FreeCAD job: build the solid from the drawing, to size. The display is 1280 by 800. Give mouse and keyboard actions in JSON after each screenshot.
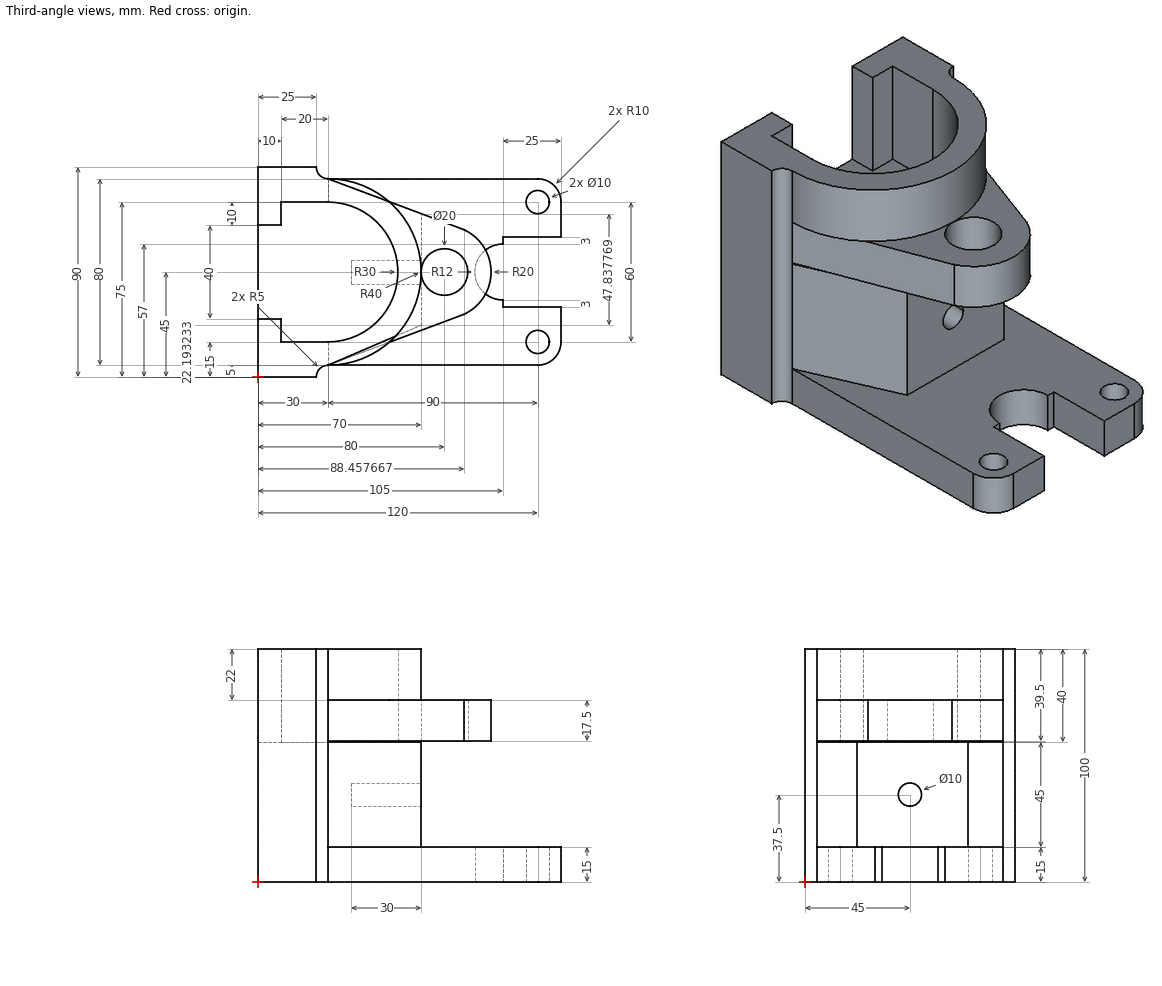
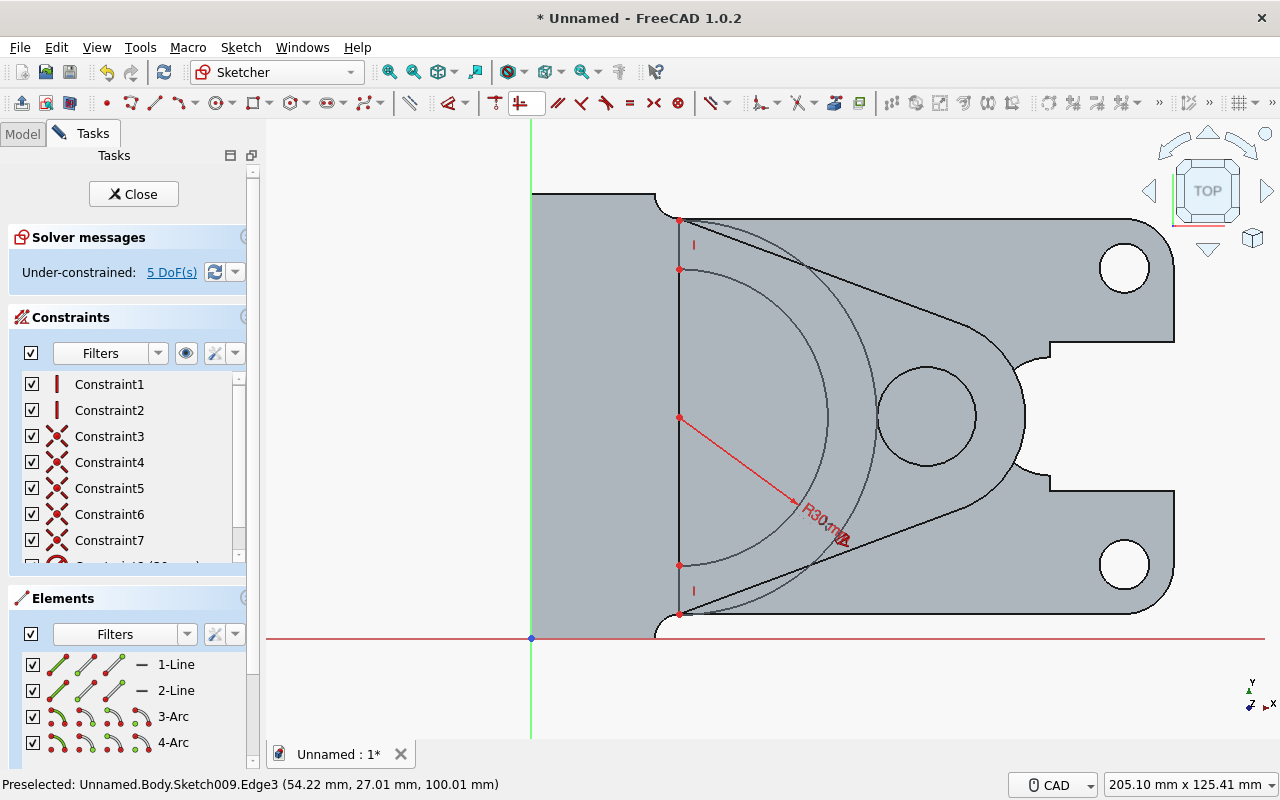
{"action": "left_click", "coordinate": [839, 534]}
{"action": "left_click", "coordinate": [865, 553]}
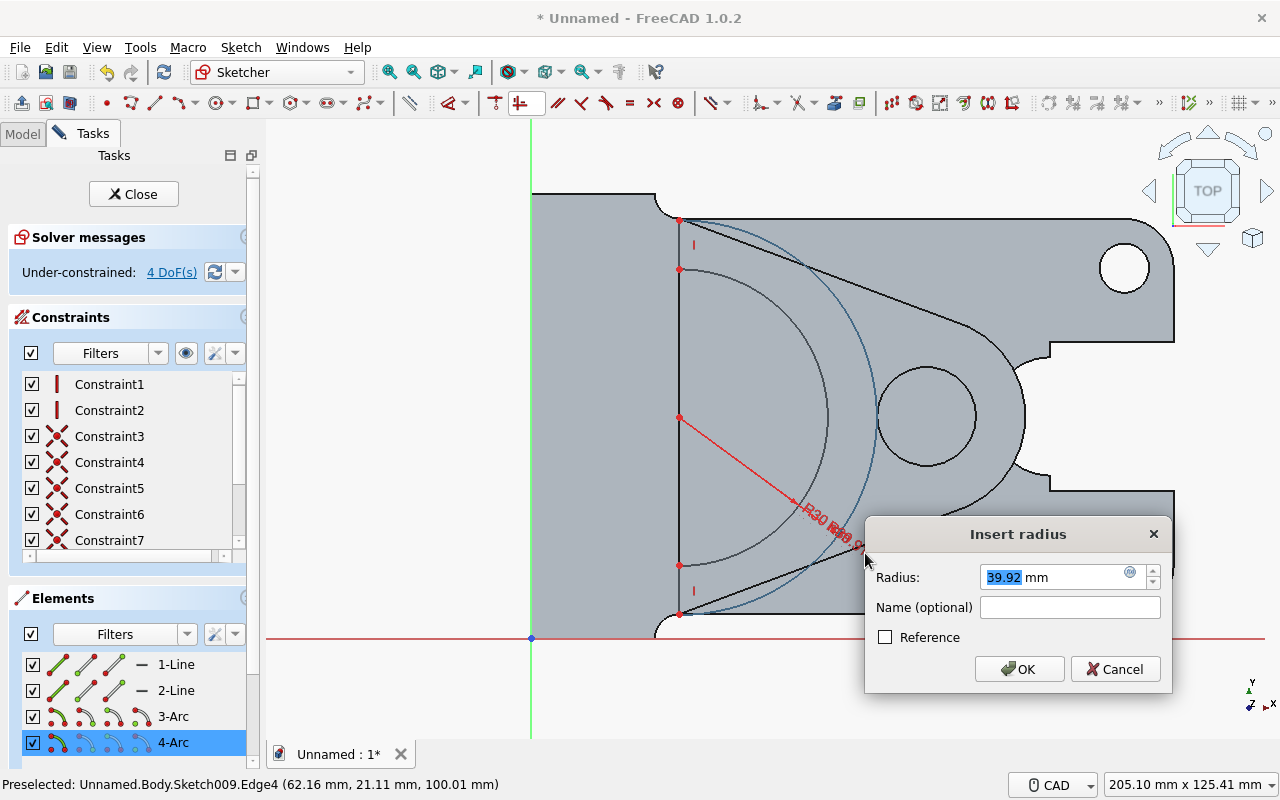
{"action": "type", "text": "40"}
{"action": "key", "text": "Return"}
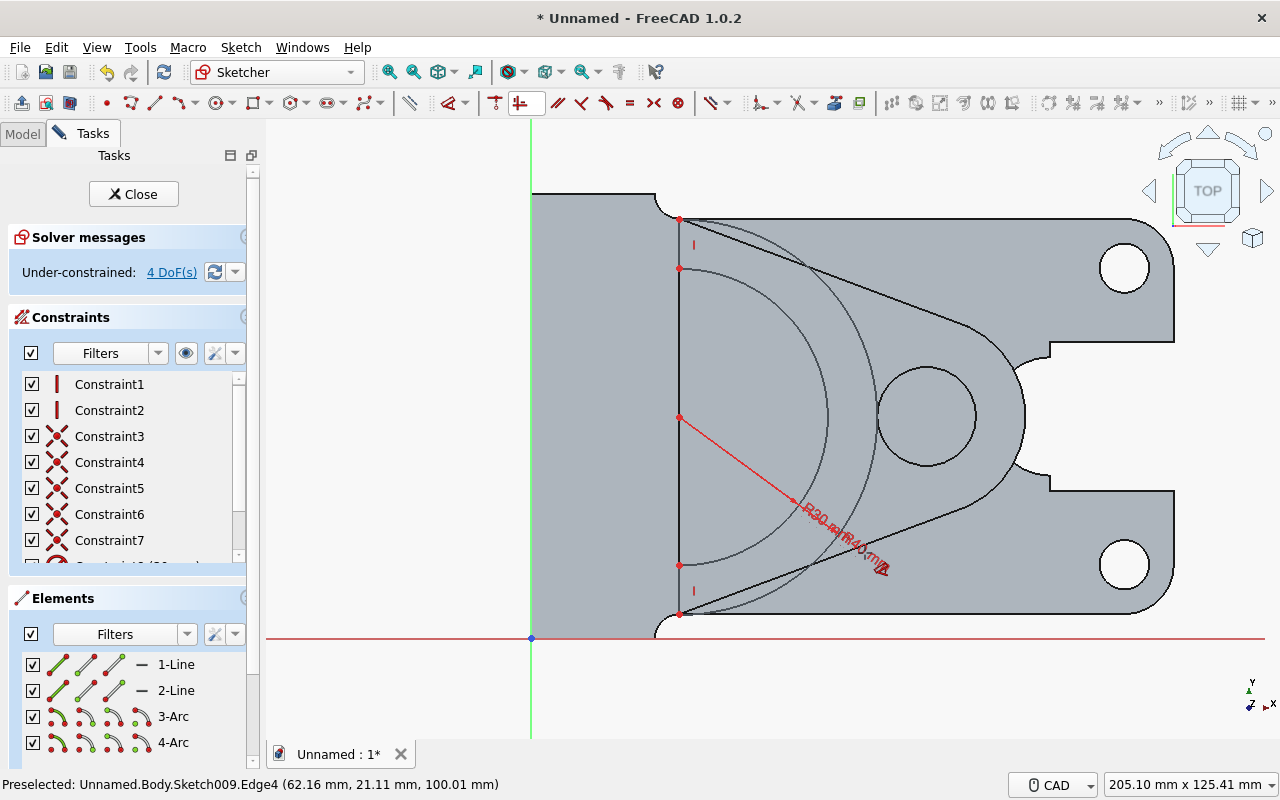
{"action": "scroll", "coordinate": [679, 615], "scroll_direction": "up", "scroll_amount": 3}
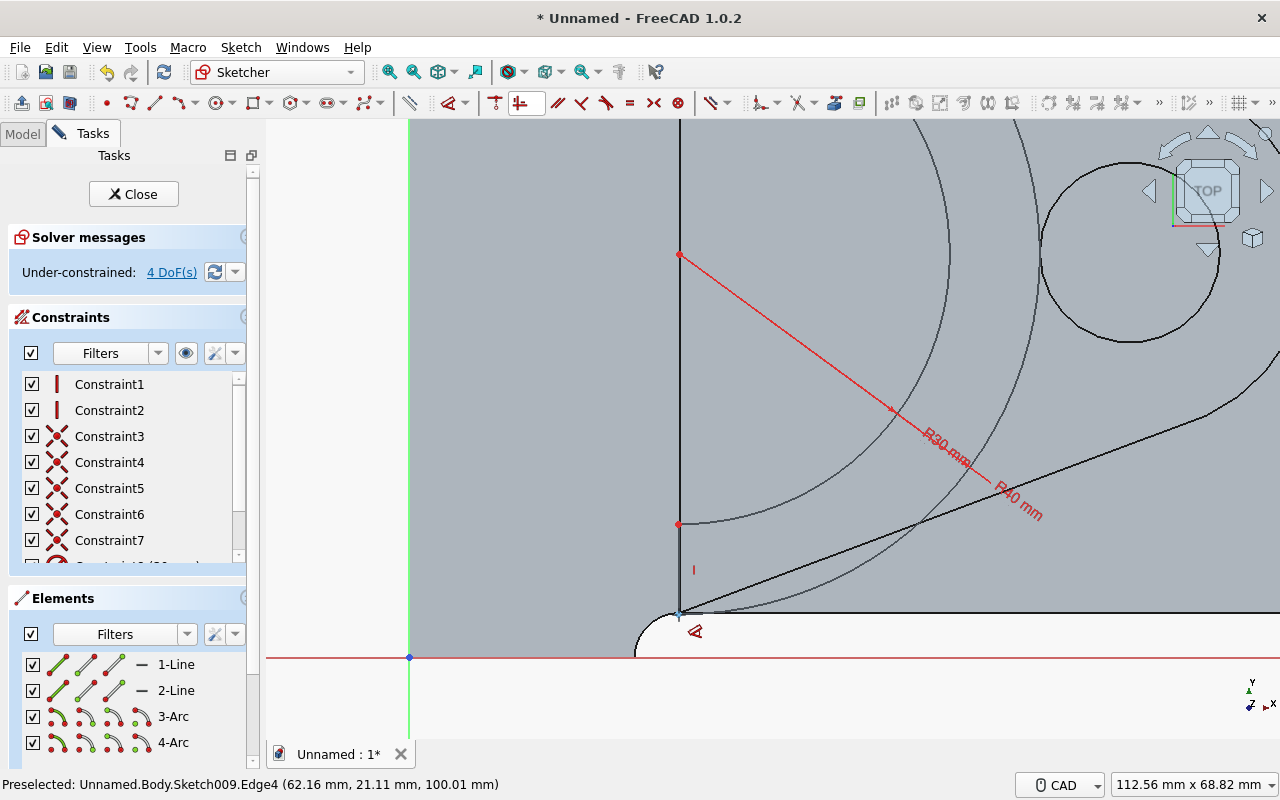
{"action": "left_click", "coordinate": [679, 614]}
{"action": "left_click", "coordinate": [375, 636]}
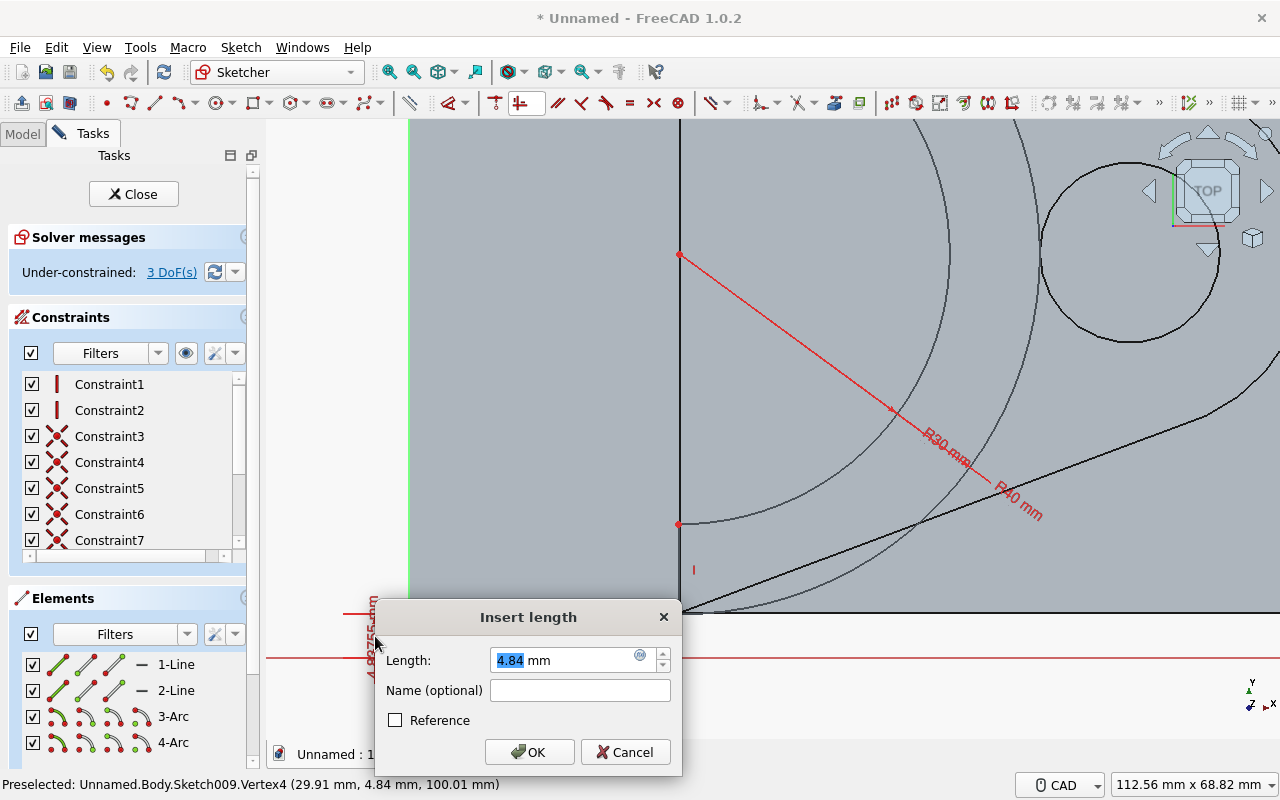
{"action": "type", "text": "5"}
{"action": "key", "text": "Return"}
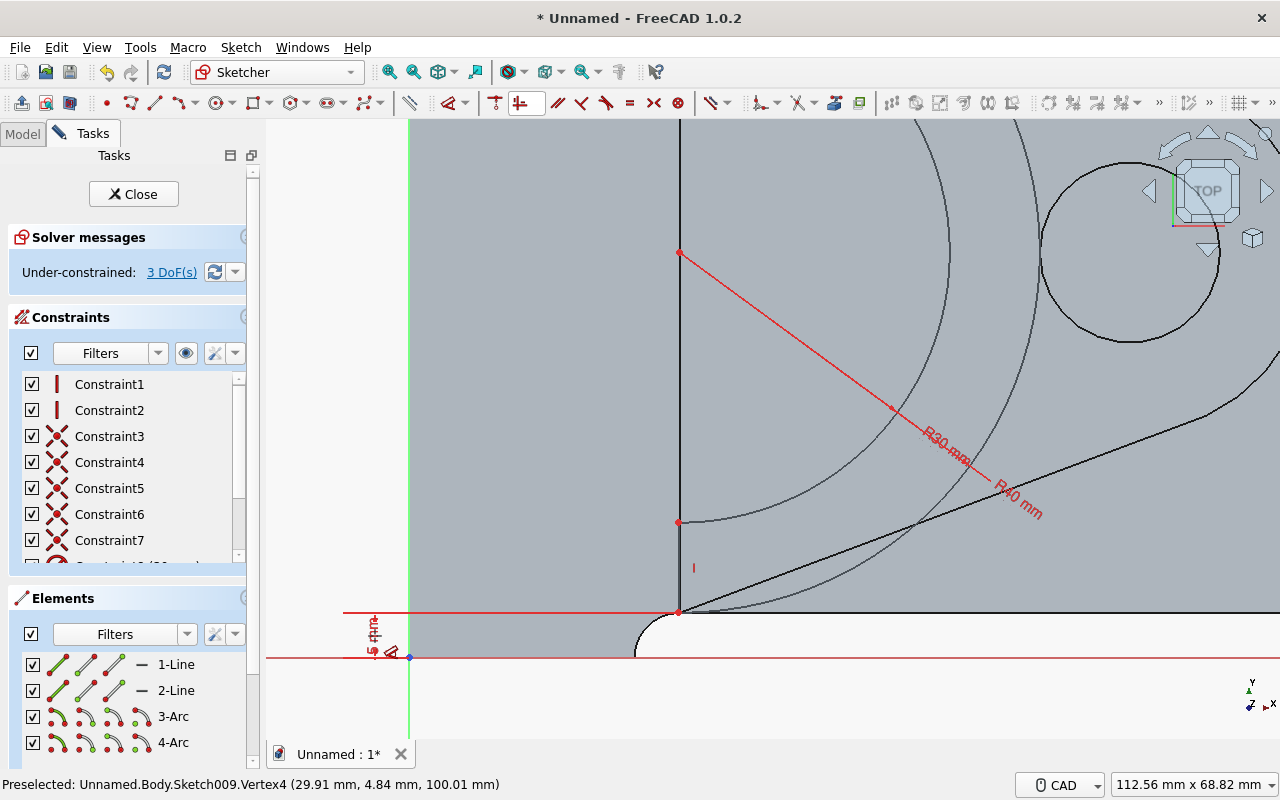
{"action": "scroll", "coordinate": [680, 616], "scroll_direction": "down", "scroll_amount": 3}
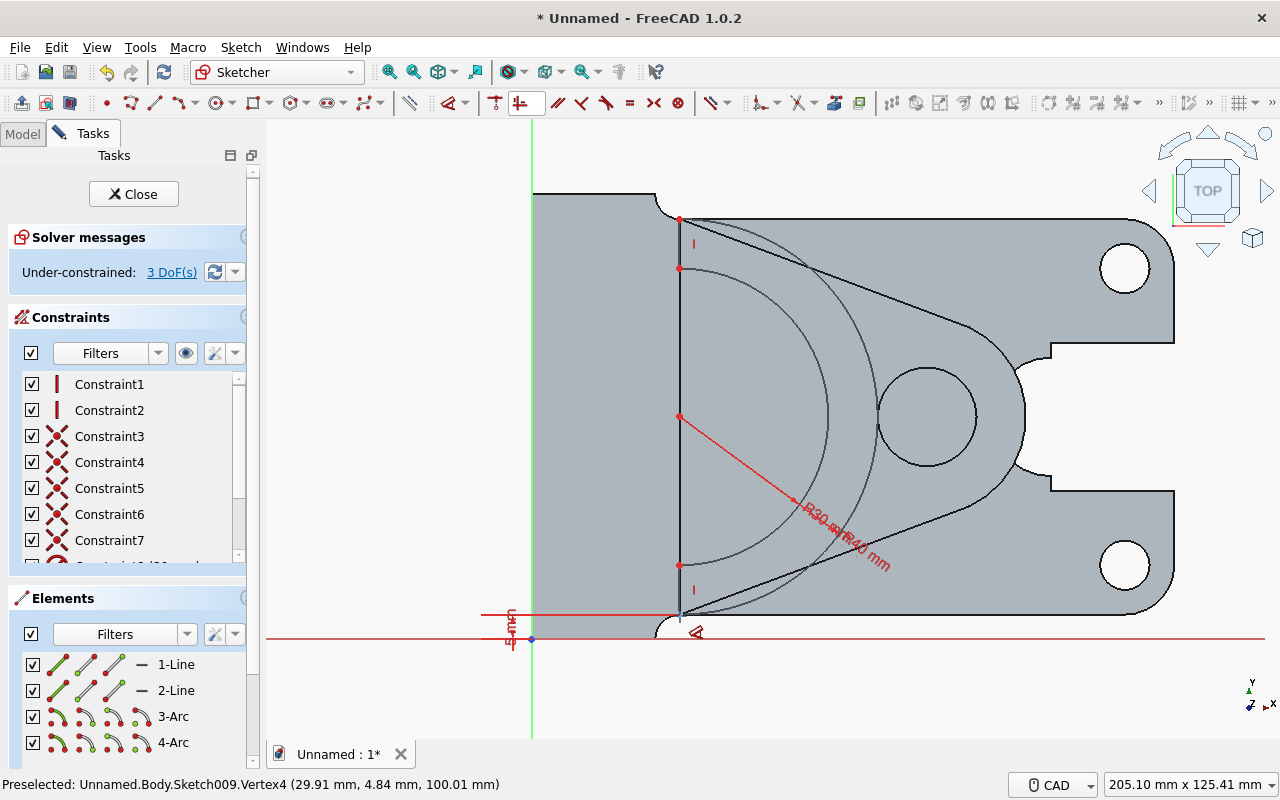
{"action": "left_click", "coordinate": [679, 219]}
{"action": "left_click", "coordinate": [606, 673]}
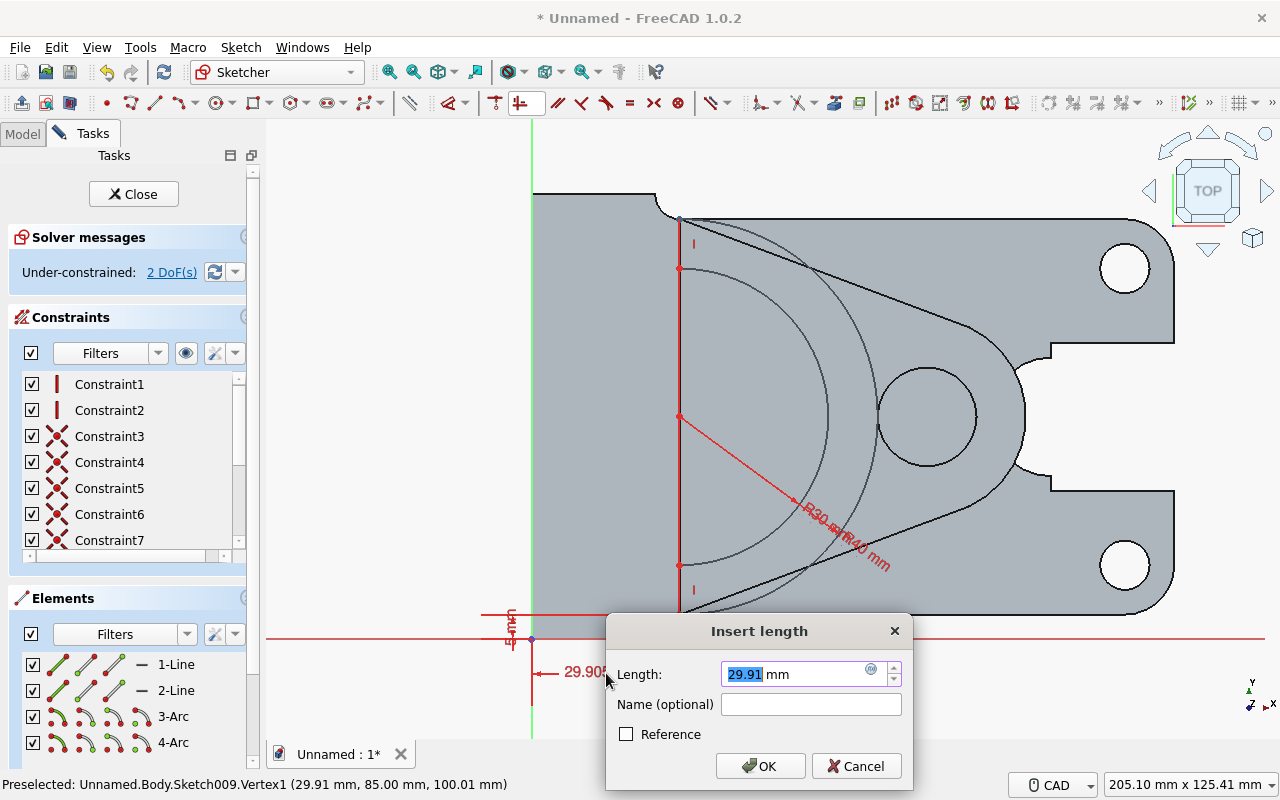
{"action": "type", "text": "30"}
{"action": "key", "text": "Return"}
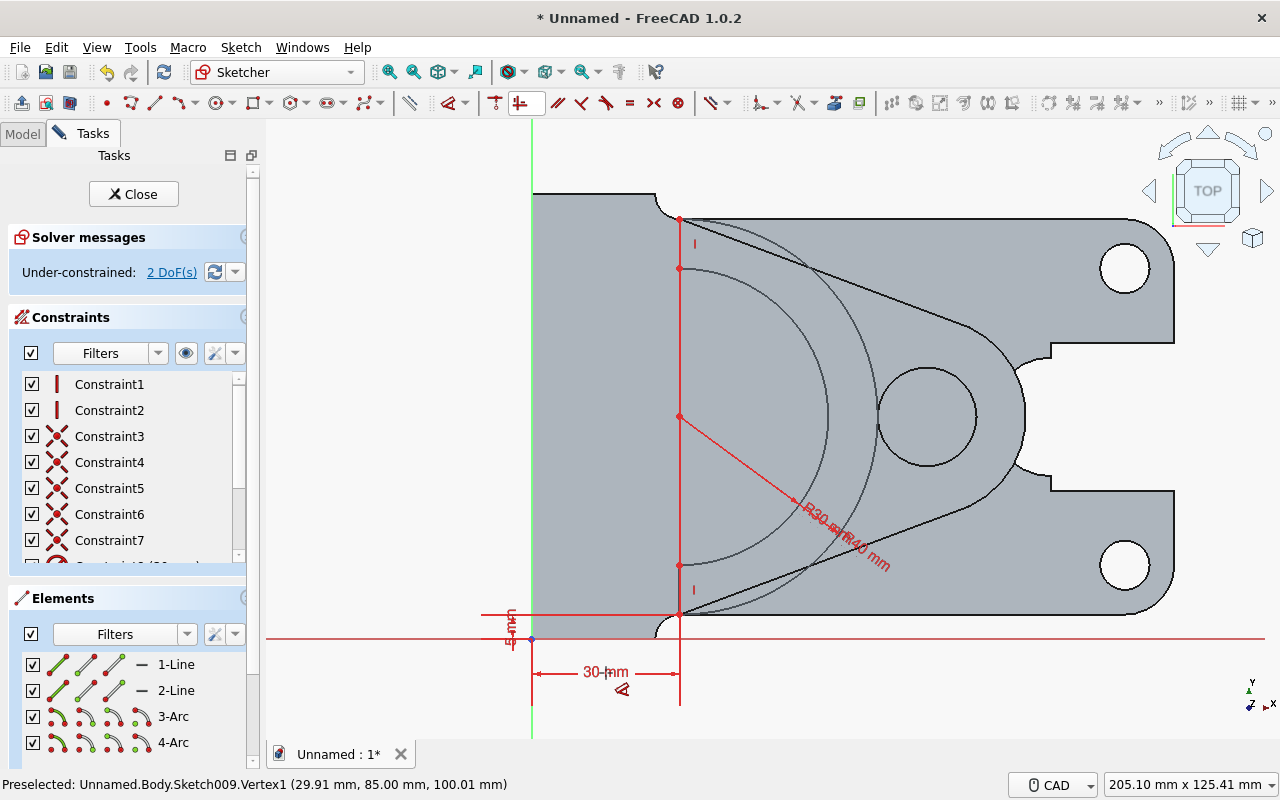
{"action": "left_click", "coordinate": [679, 565]}
{"action": "left_click", "coordinate": [606, 531]}